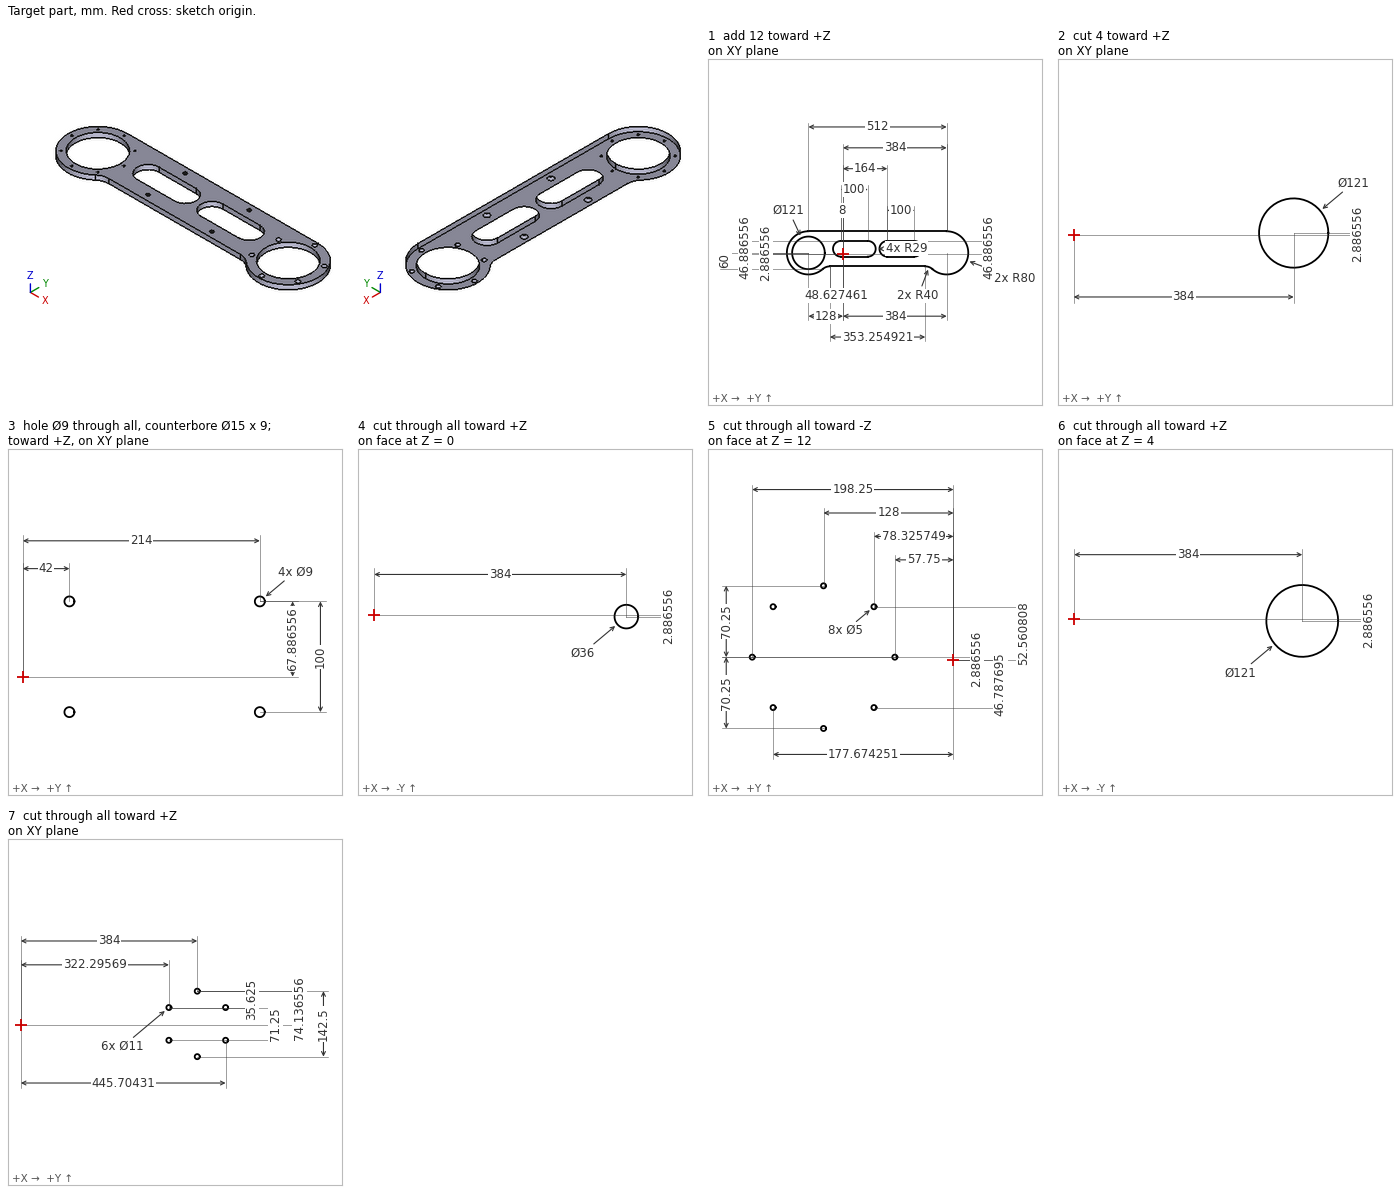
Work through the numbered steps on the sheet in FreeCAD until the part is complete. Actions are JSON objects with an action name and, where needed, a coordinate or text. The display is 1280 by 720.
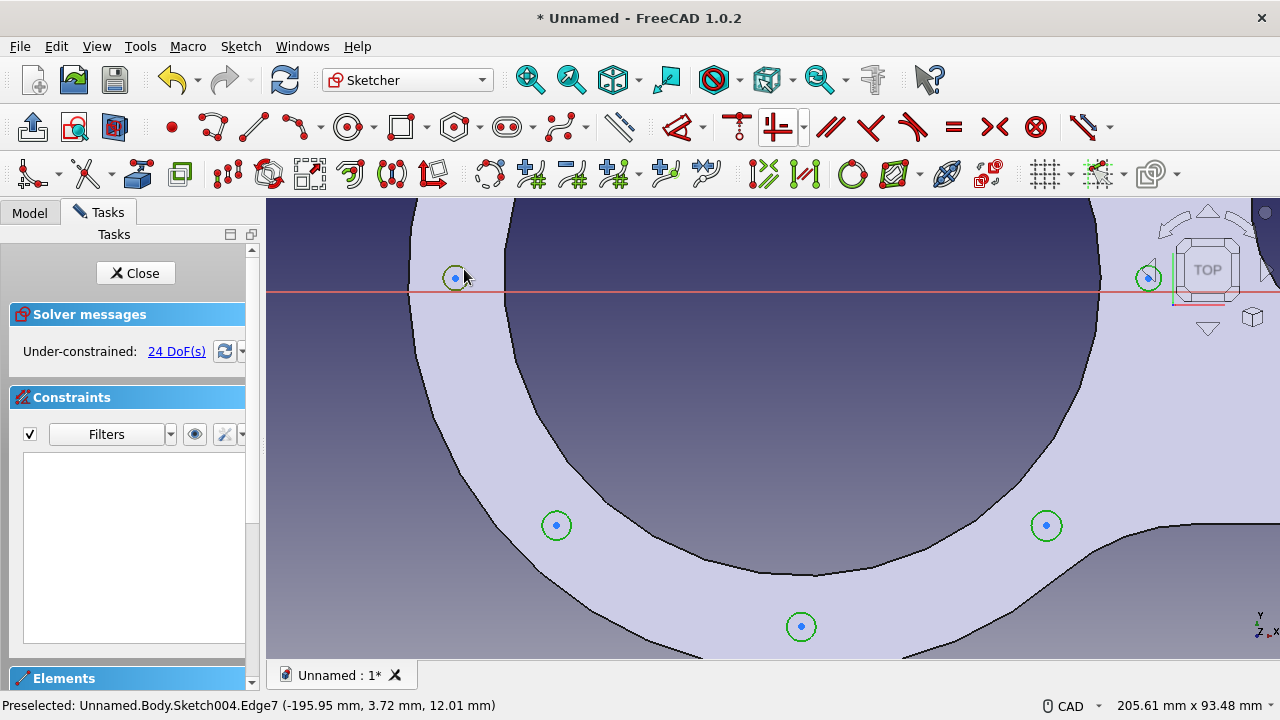
{"action": "scroll", "coordinate": [568, 516], "scroll_direction": "down", "scroll_amount": 5}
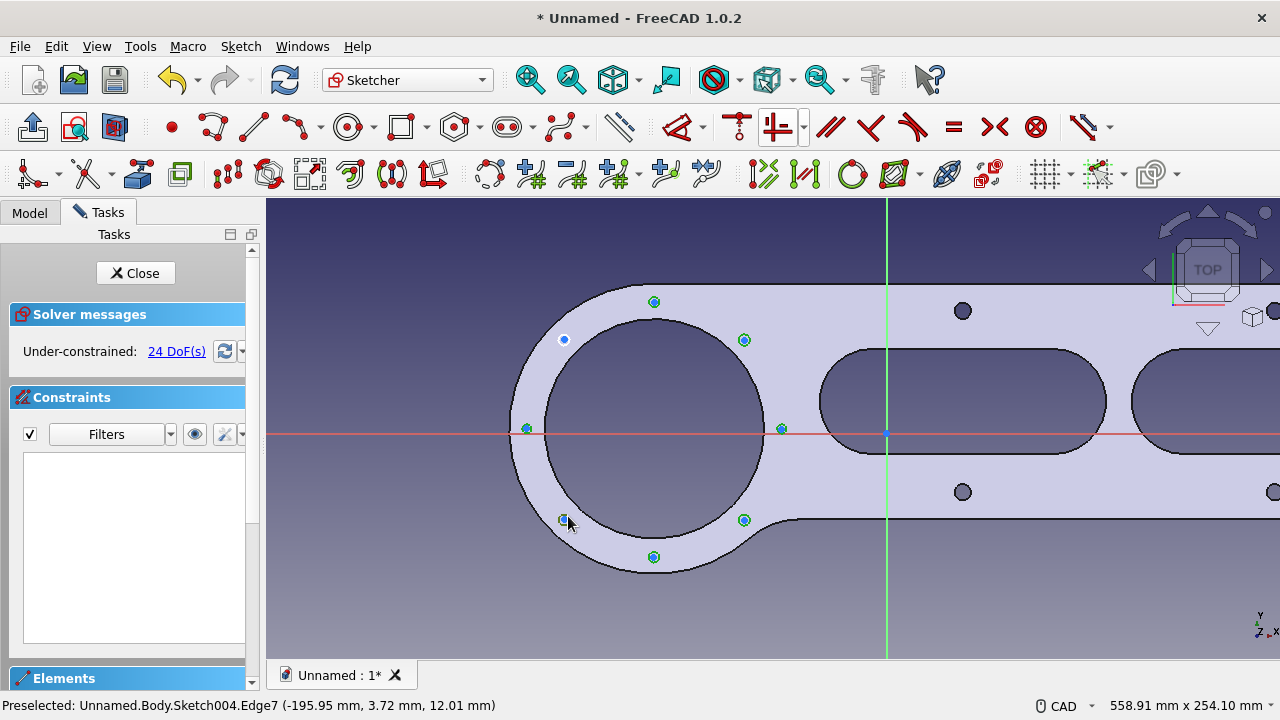
{"action": "scroll", "coordinate": [568, 336], "scroll_direction": "up", "scroll_amount": 5}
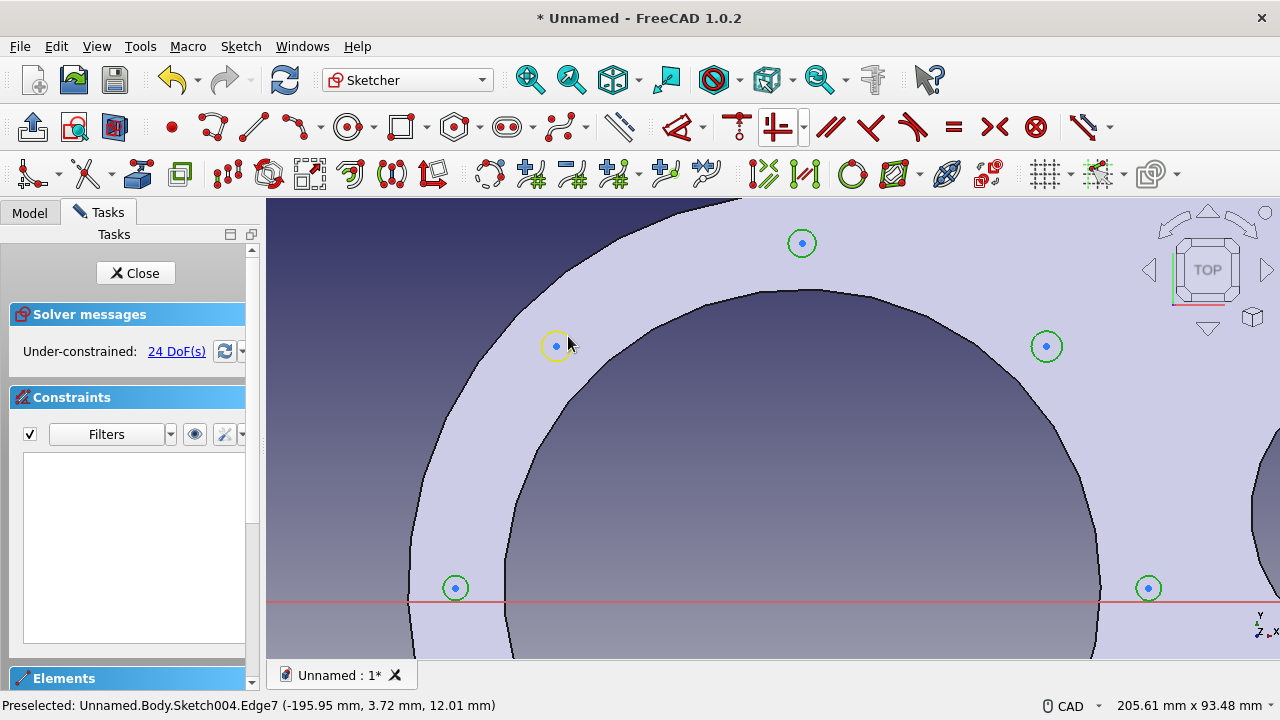
{"action": "left_click", "coordinate": [567, 336]}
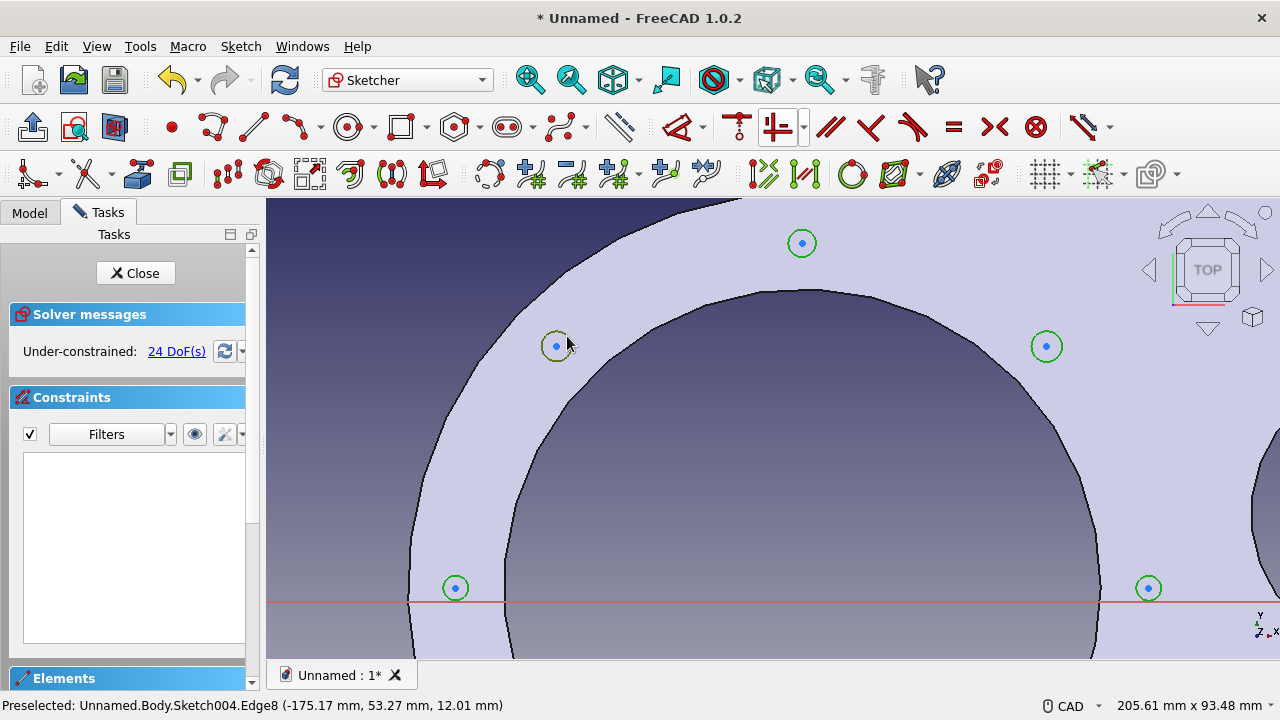
{"action": "left_click", "coordinate": [954, 128]}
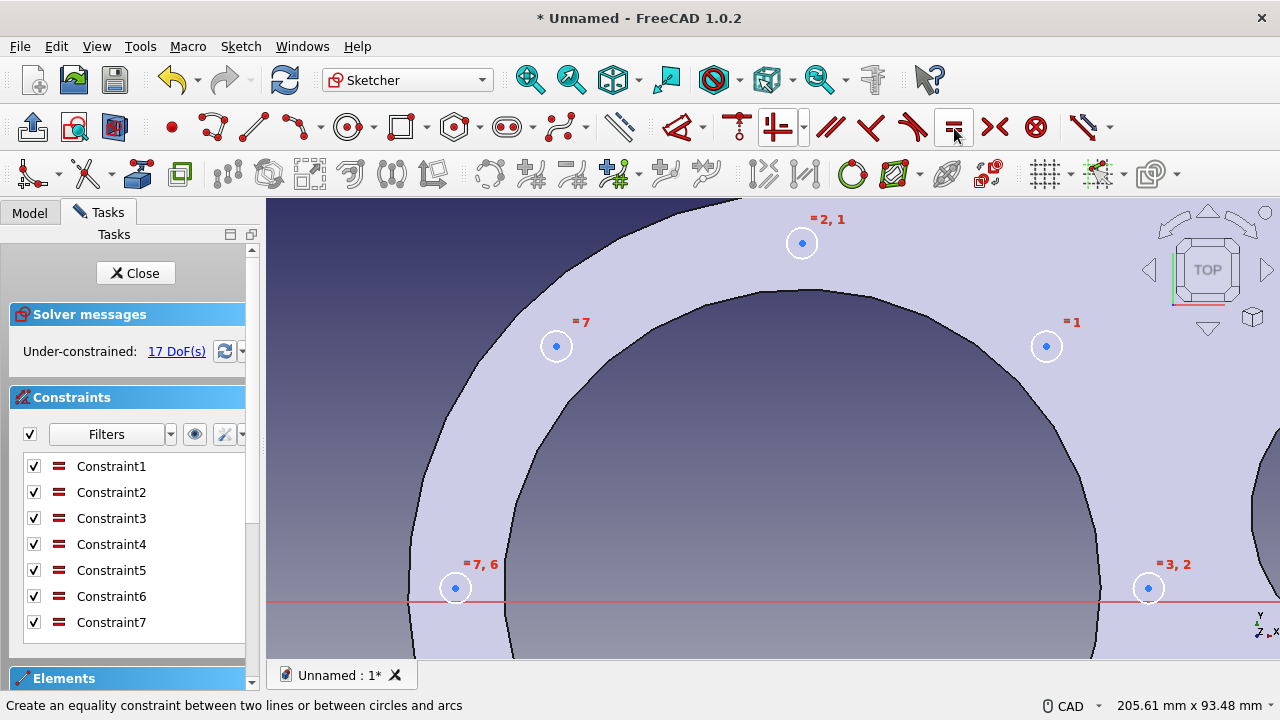
{"action": "left_click", "coordinate": [1047, 347]}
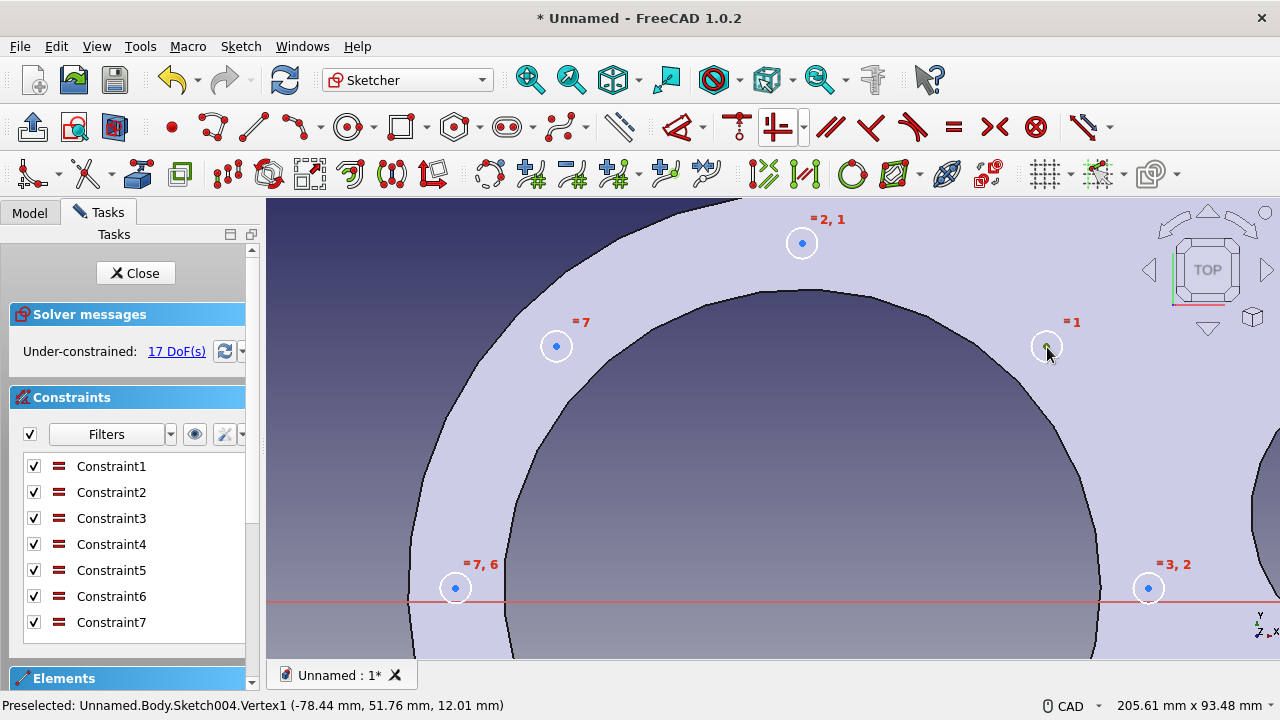
{"action": "scroll", "coordinate": [568, 336], "scroll_direction": "down", "scroll_amount": 5}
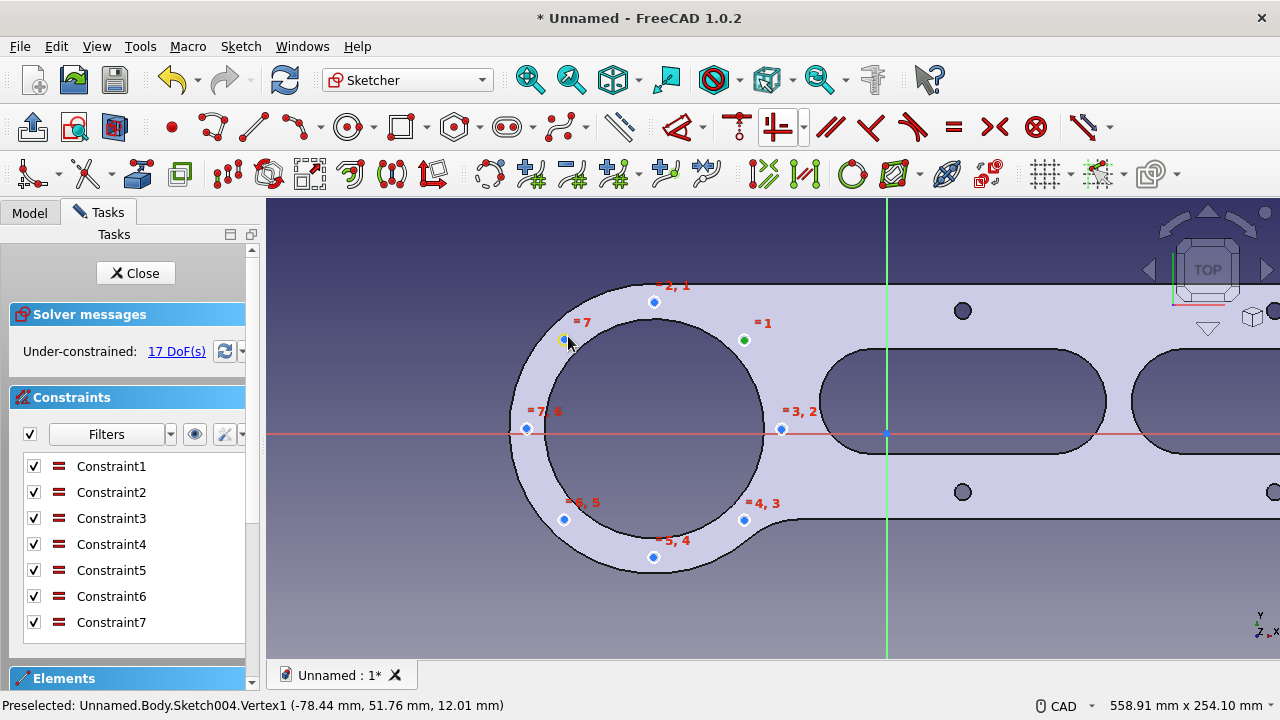
{"action": "left_click", "coordinate": [744, 520]}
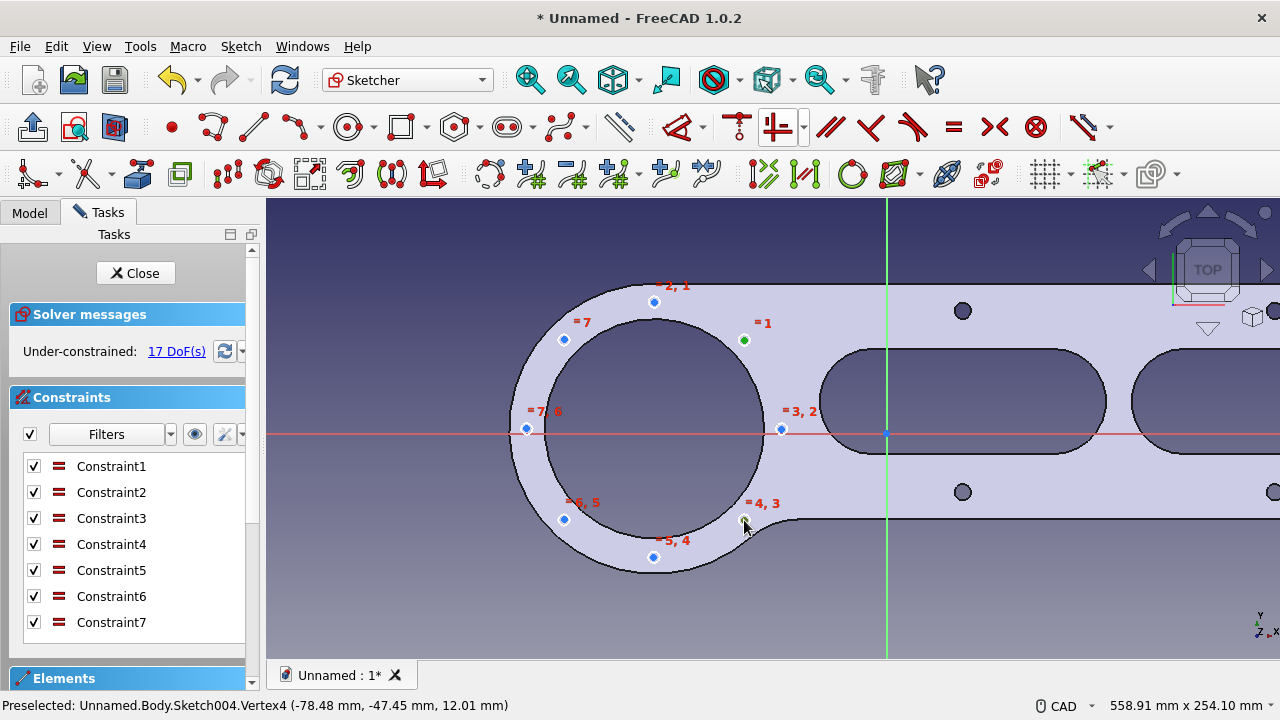
{"action": "key", "text": "v"}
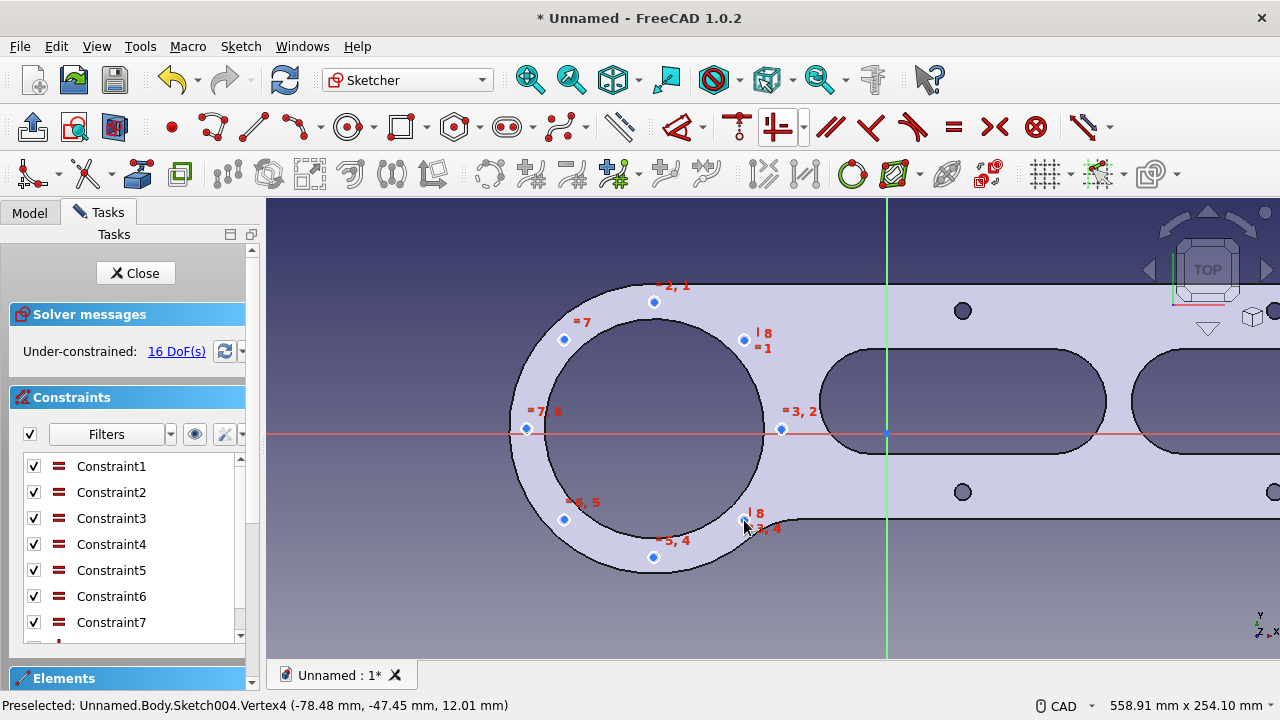
{"action": "left_click", "coordinate": [654, 302]}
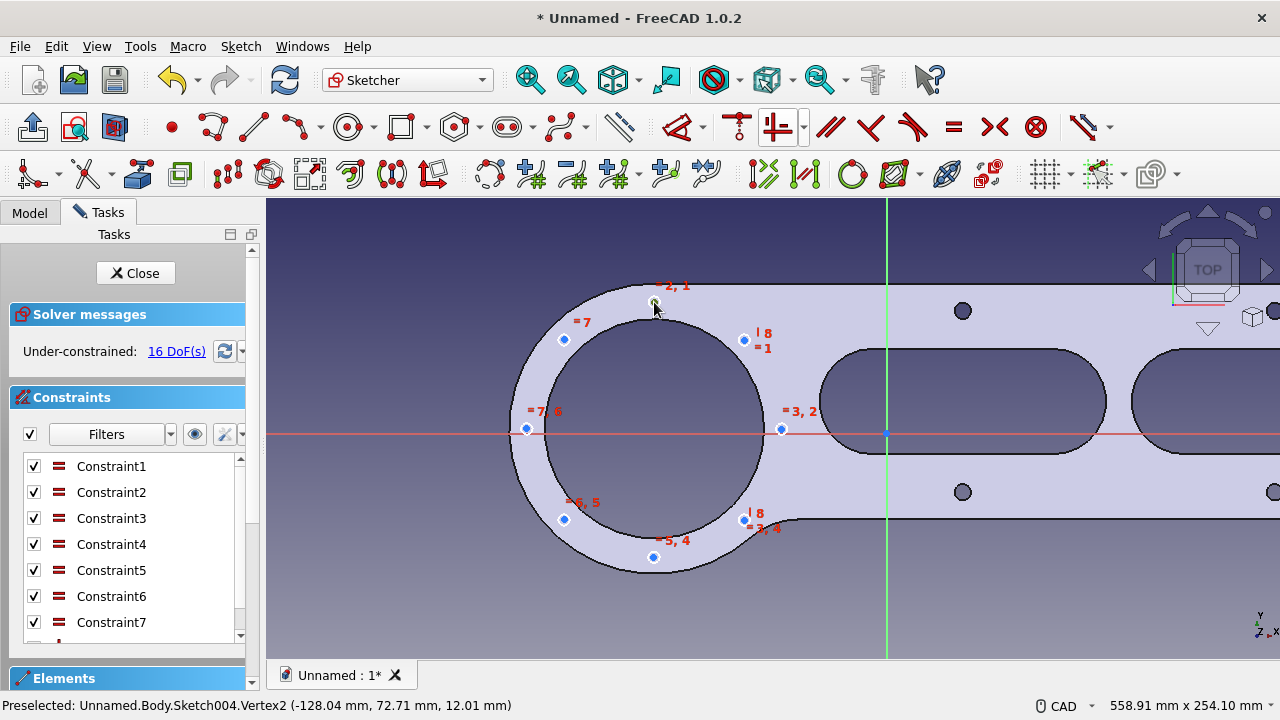
{"action": "left_click", "coordinate": [654, 557]}